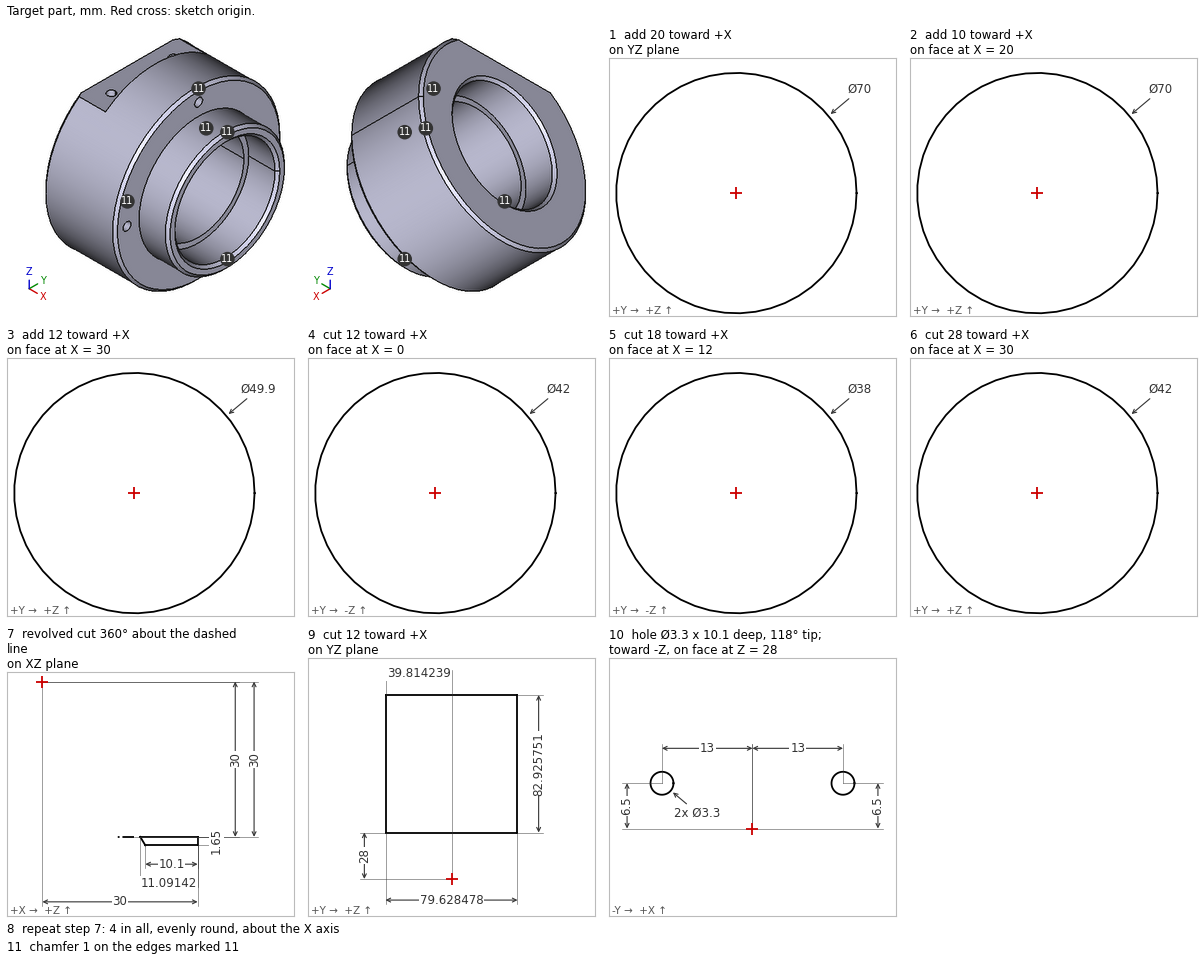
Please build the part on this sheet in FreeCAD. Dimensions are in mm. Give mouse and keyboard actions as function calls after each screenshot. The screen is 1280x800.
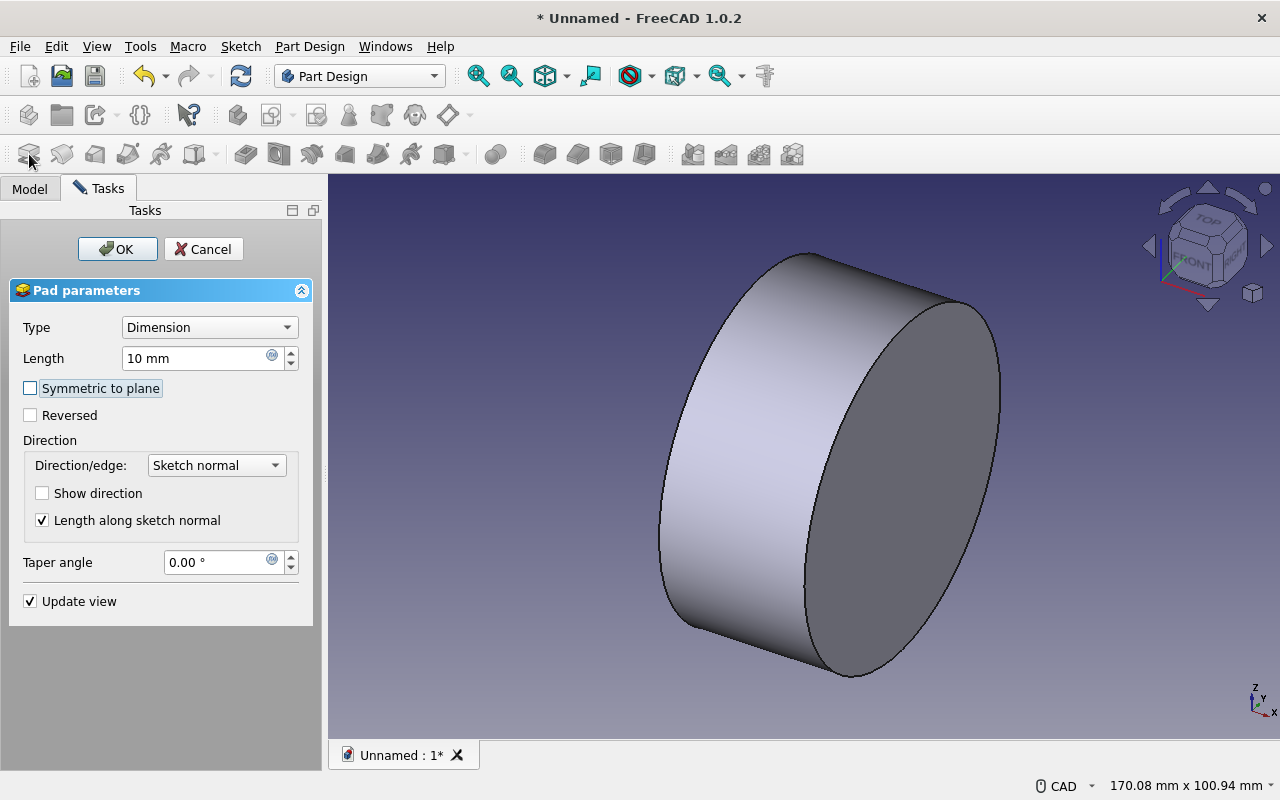
click(118, 249)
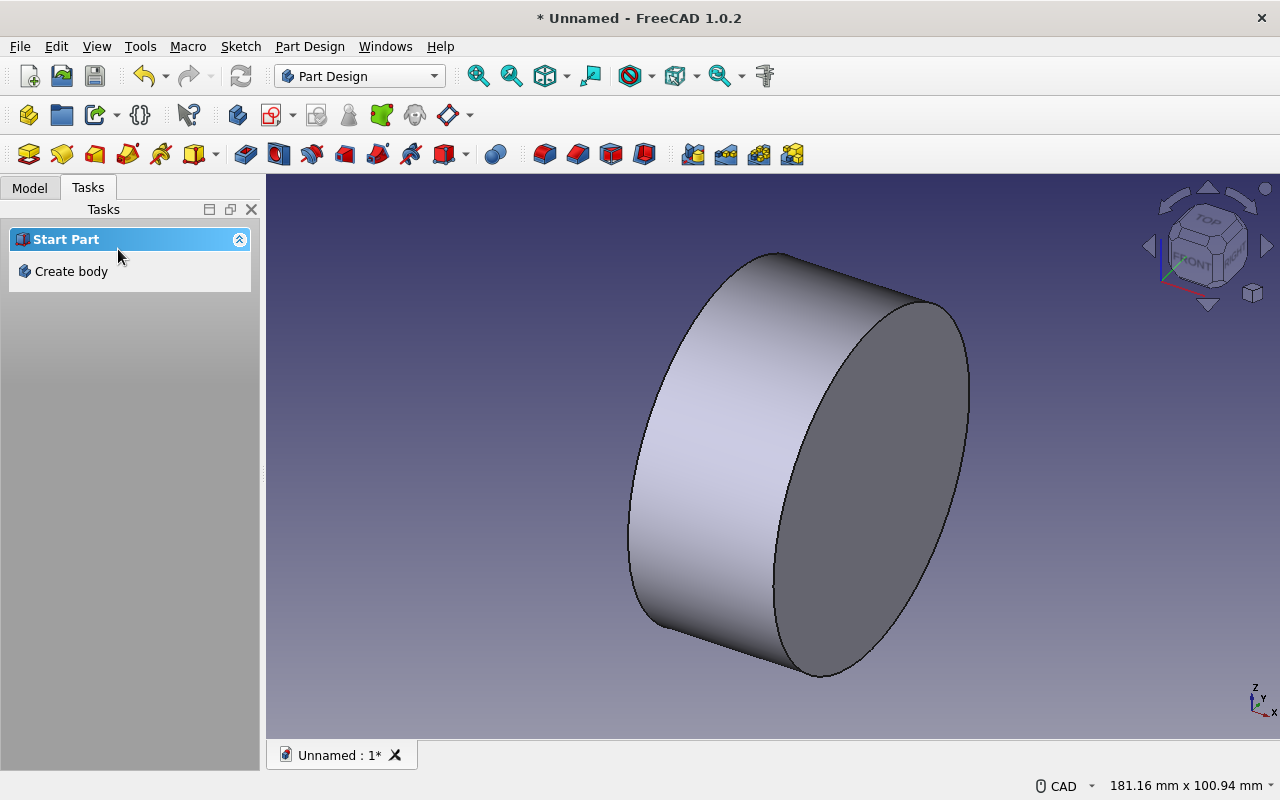
click(479, 76)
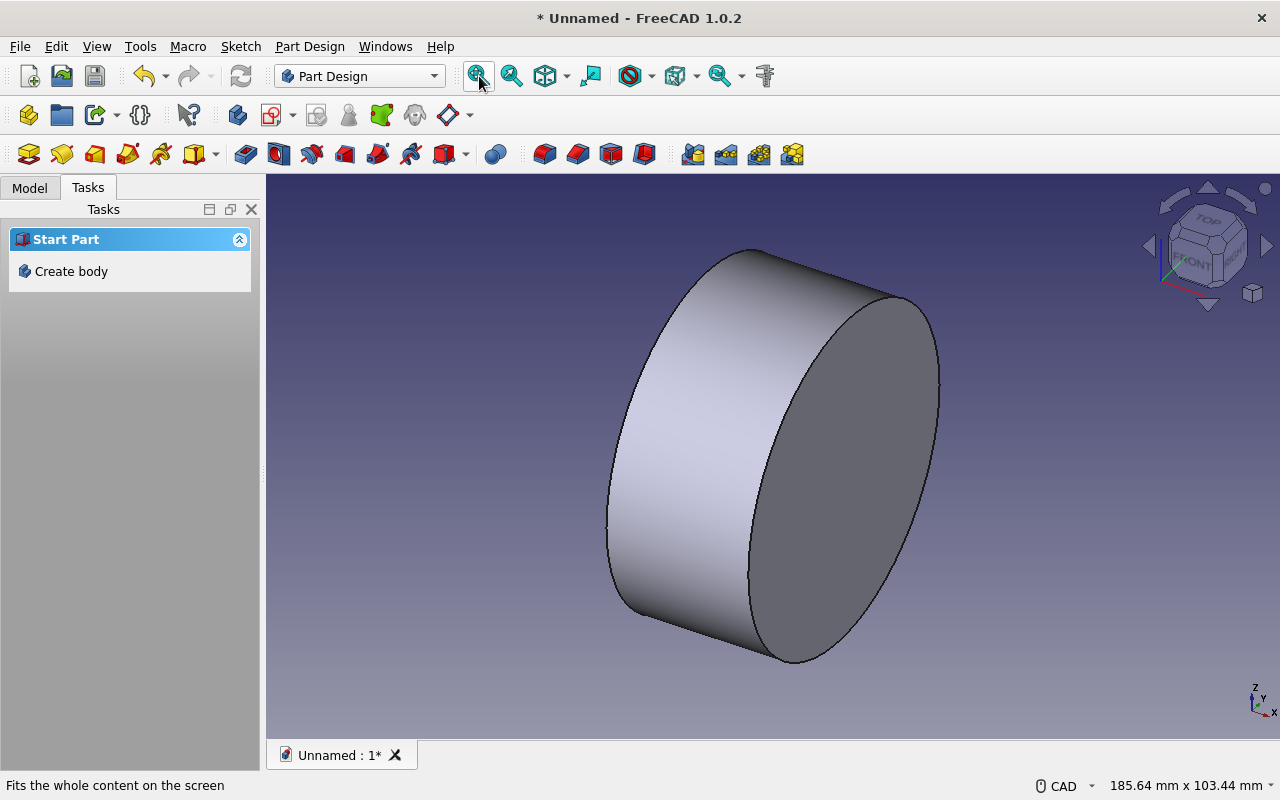
click(844, 479)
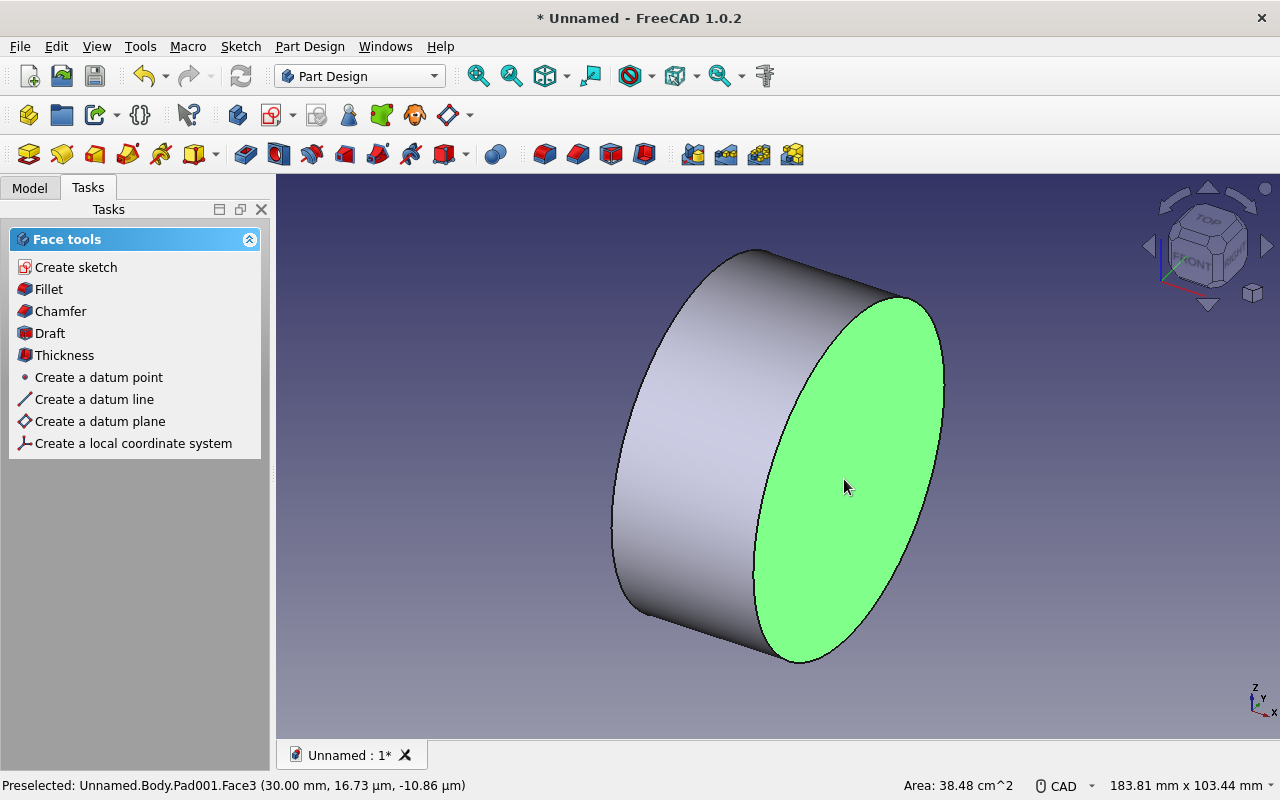
click(270, 116)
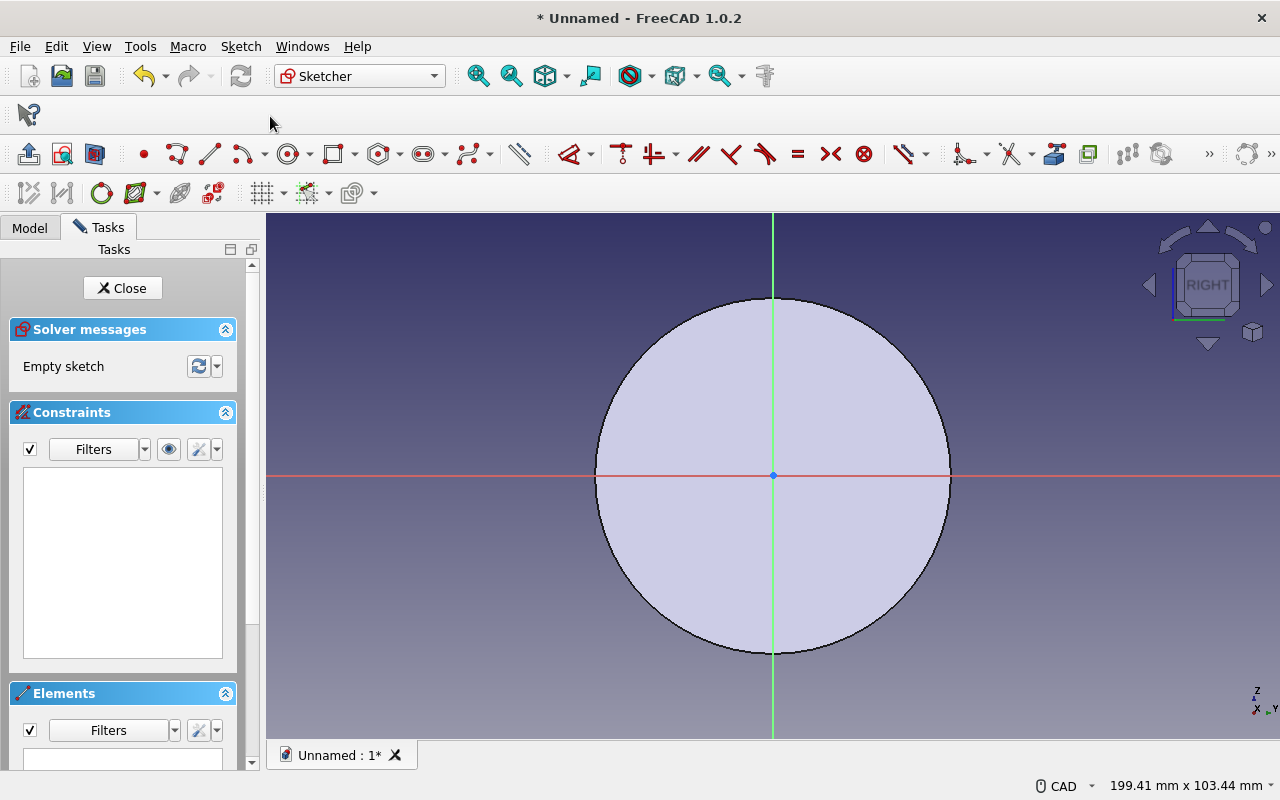
key(g)
key(c)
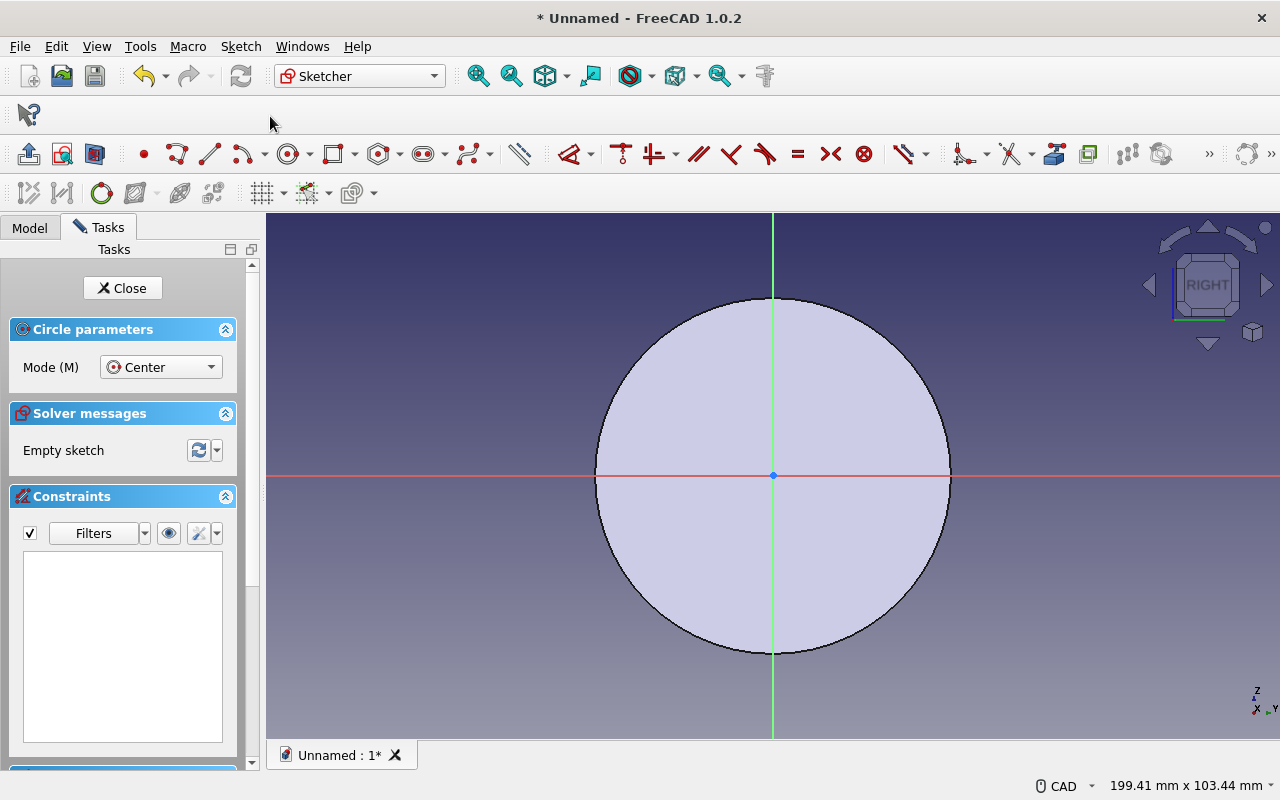
click(773, 476)
move(863, 386)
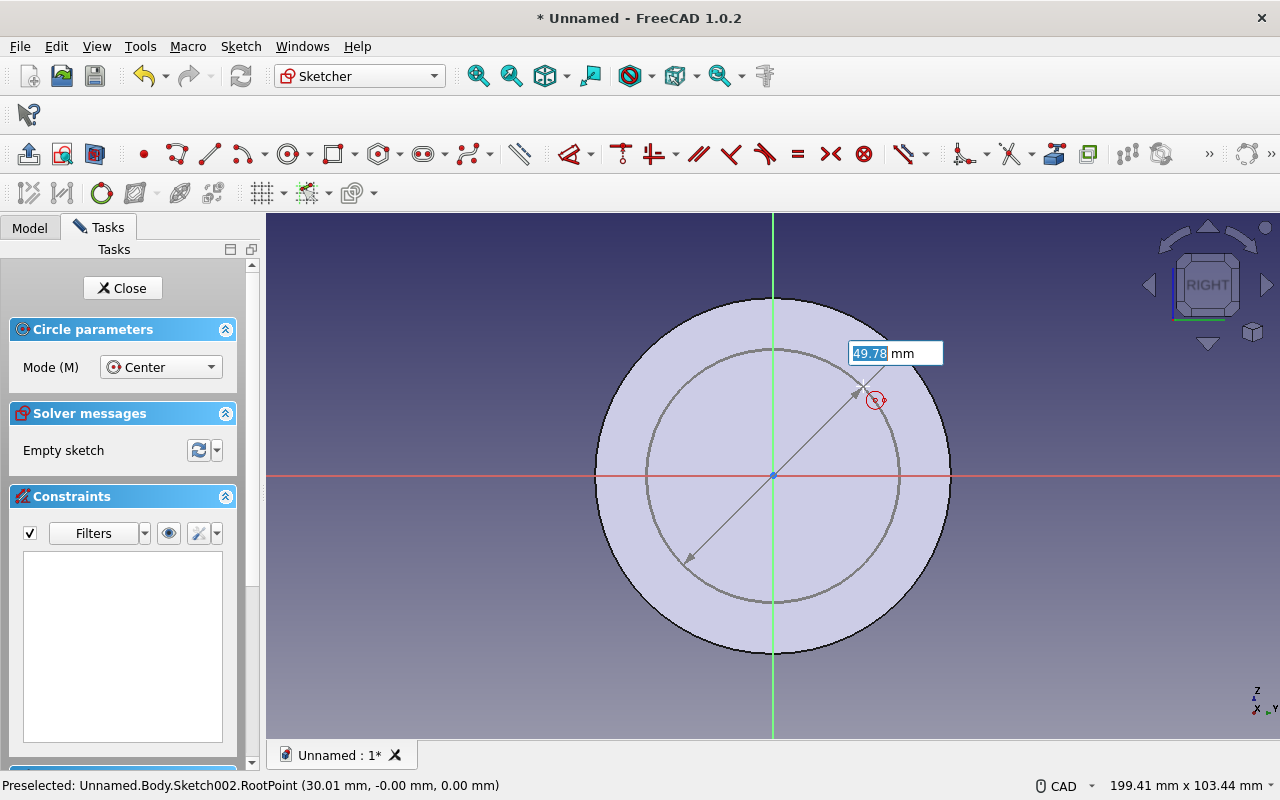
text(49.9)
key(Return)
key(Escape)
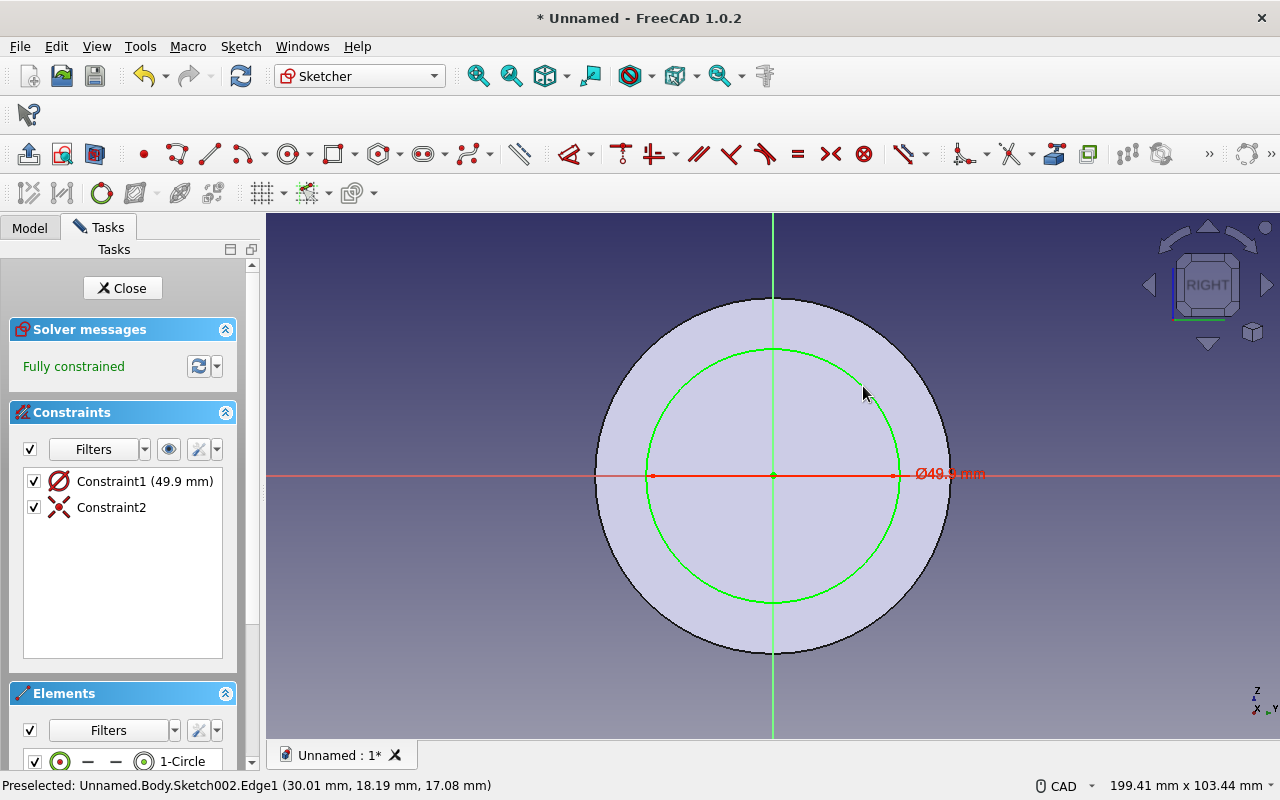
click(123, 288)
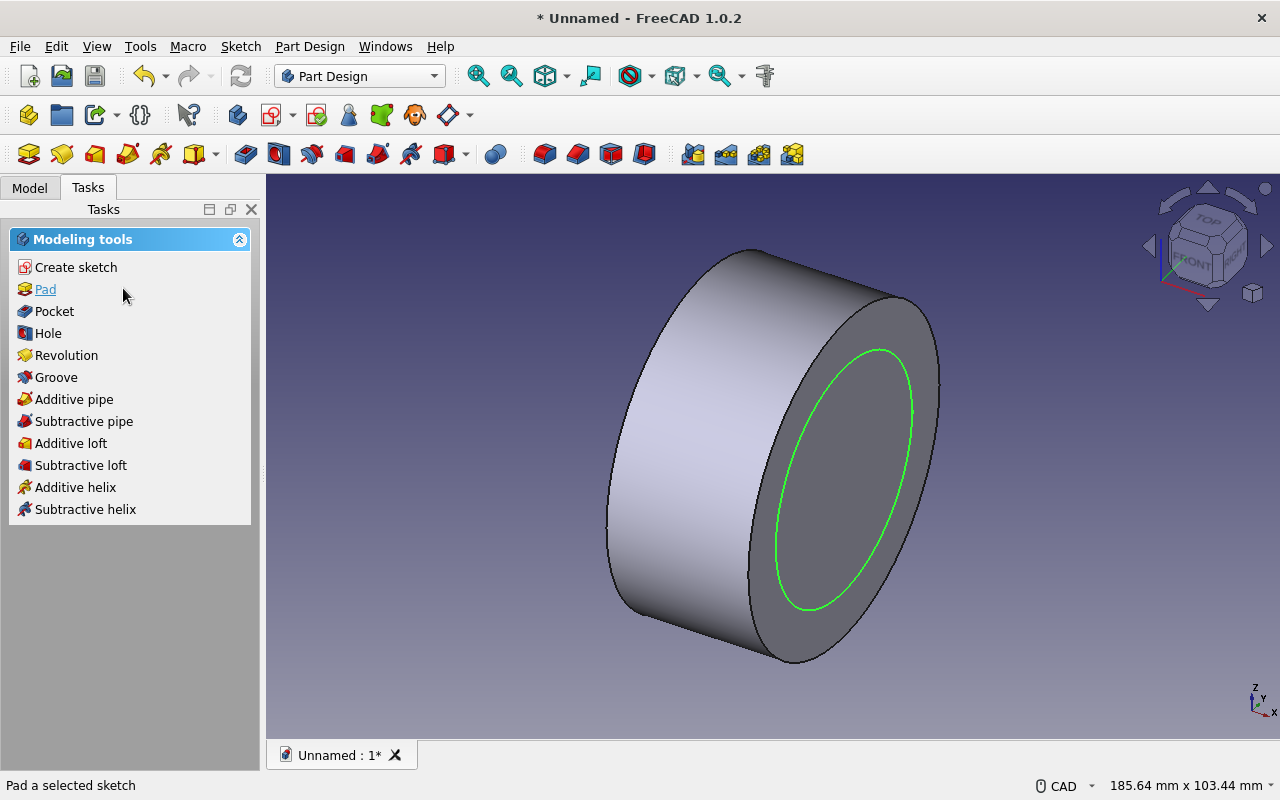
click(29, 154)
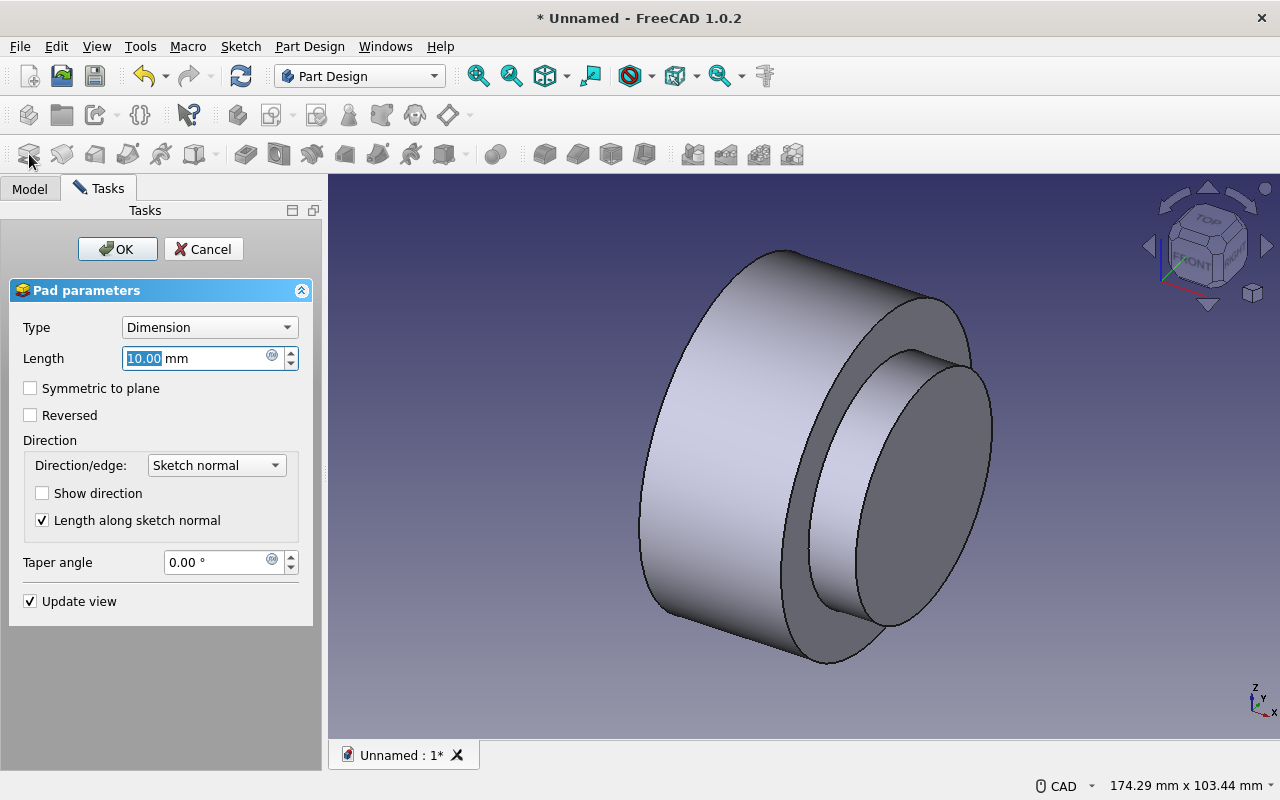
text(12)
key(Tab)